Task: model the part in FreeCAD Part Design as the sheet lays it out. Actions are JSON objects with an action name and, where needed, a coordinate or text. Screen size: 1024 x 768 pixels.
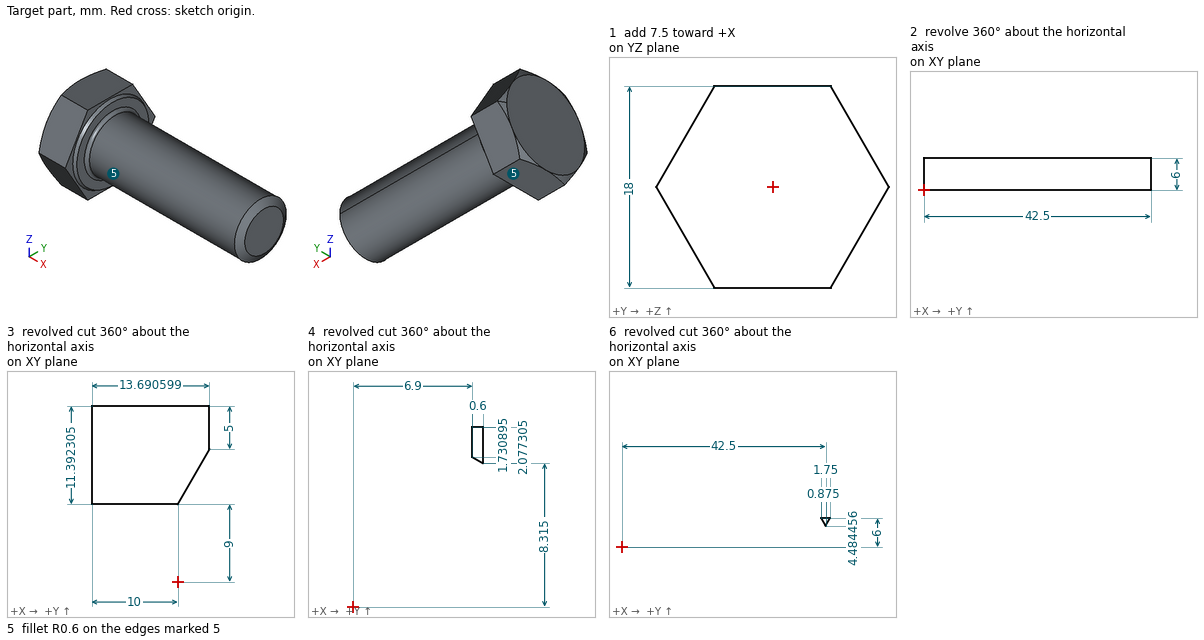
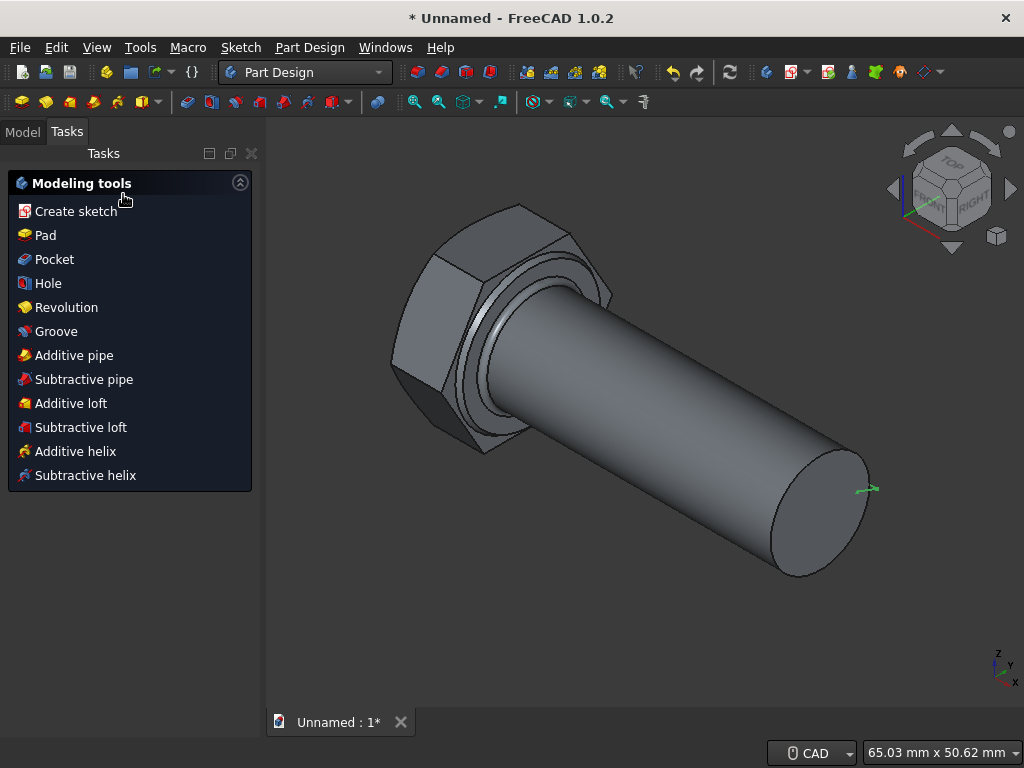
{"action": "left_click", "coordinate": [236, 102]}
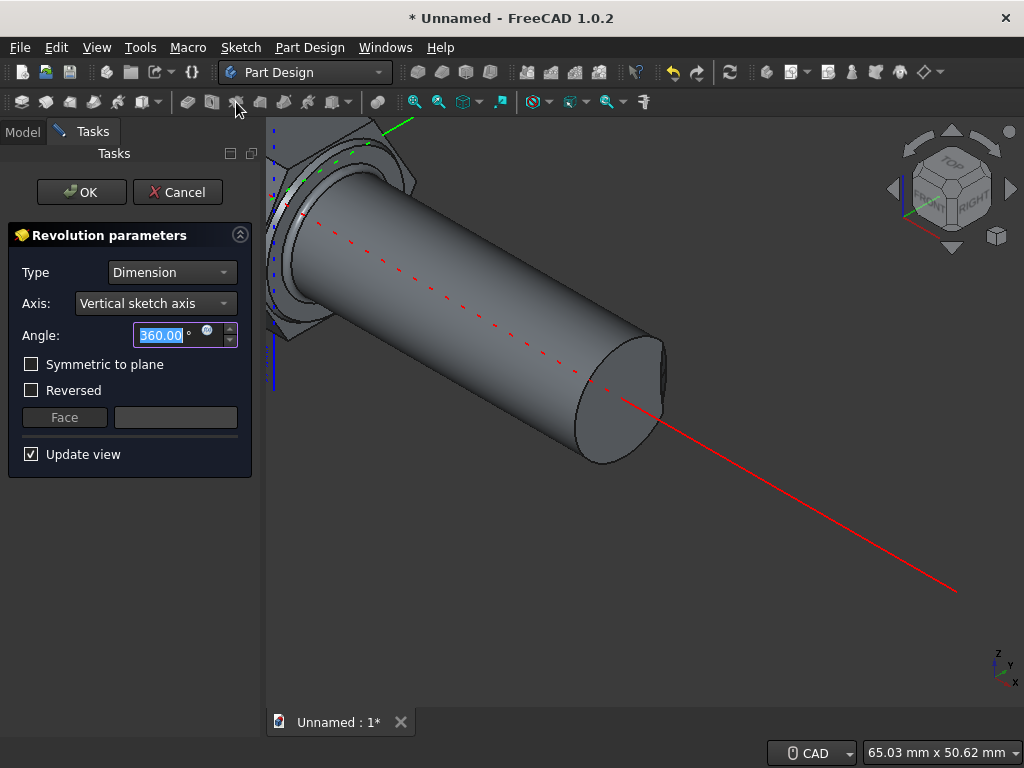
{"action": "left_click", "coordinate": [156, 304]}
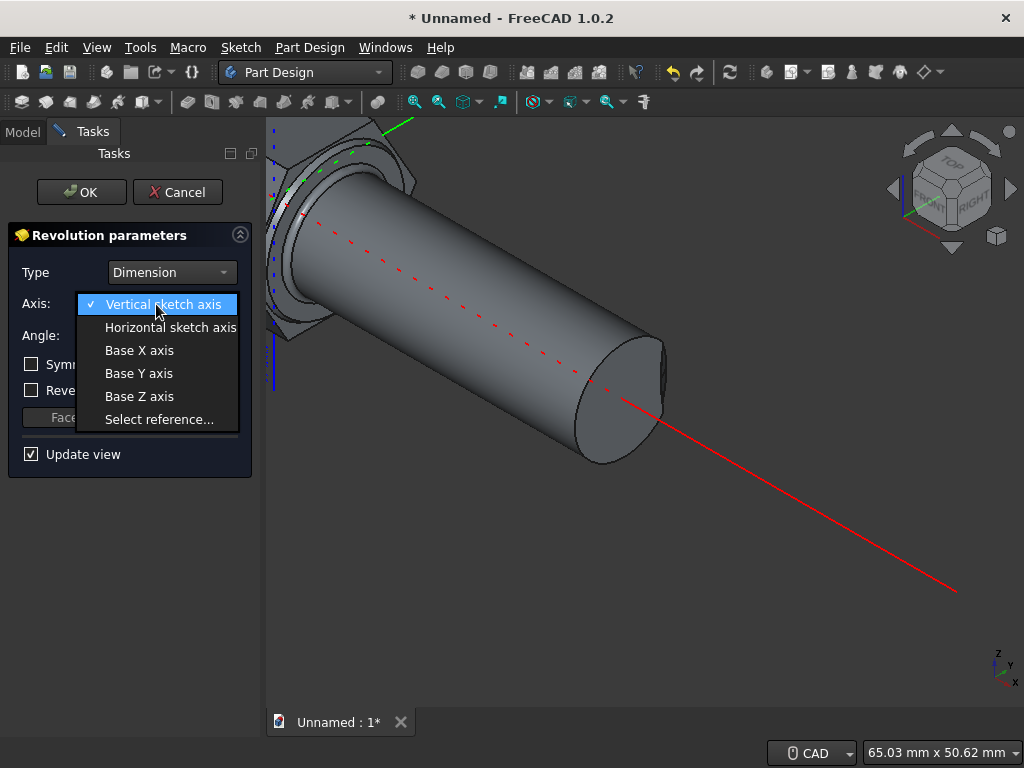
{"action": "left_click", "coordinate": [156, 328]}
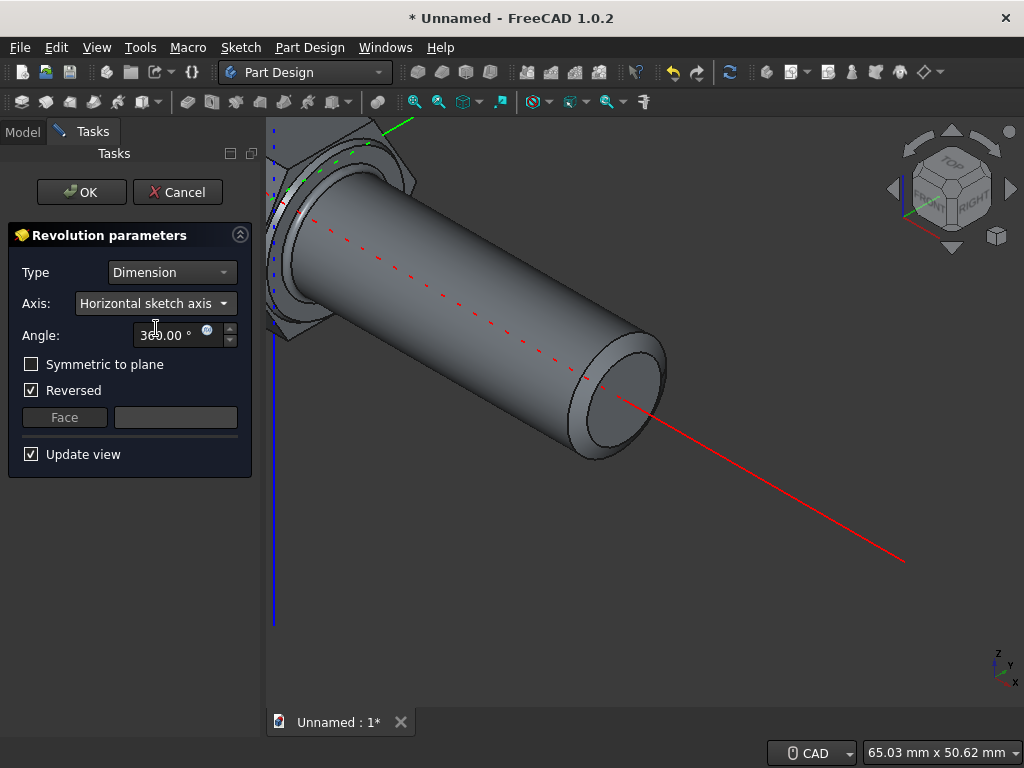
{"action": "left_click", "coordinate": [82, 192]}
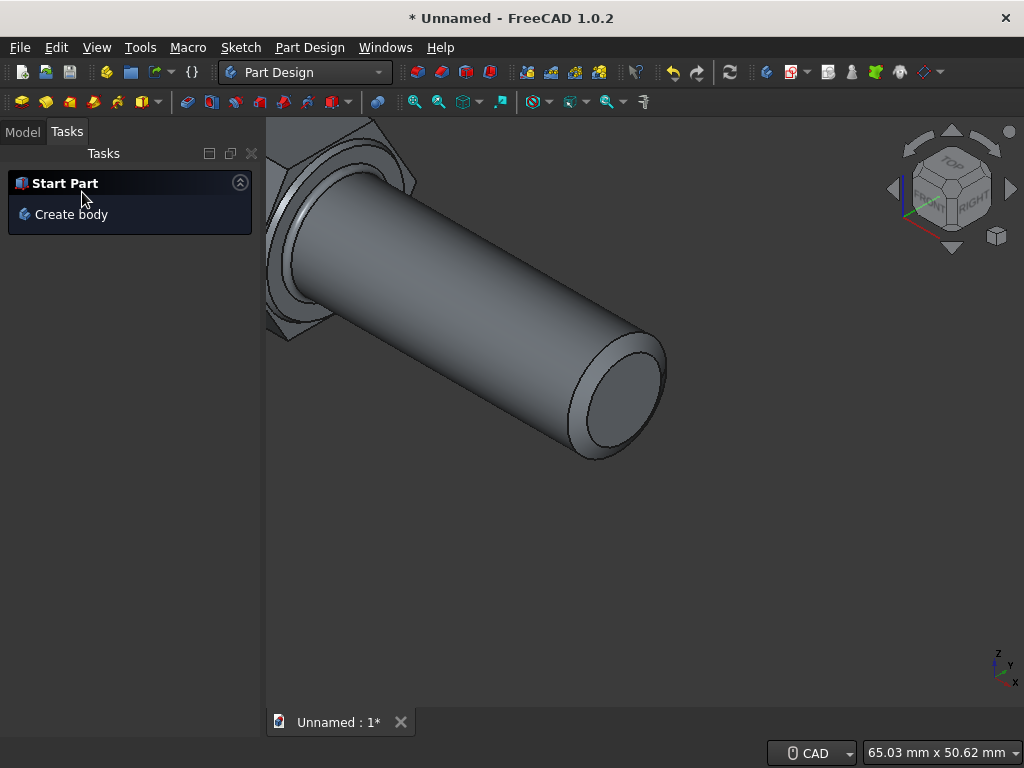
{"action": "left_click", "coordinate": [416, 102]}